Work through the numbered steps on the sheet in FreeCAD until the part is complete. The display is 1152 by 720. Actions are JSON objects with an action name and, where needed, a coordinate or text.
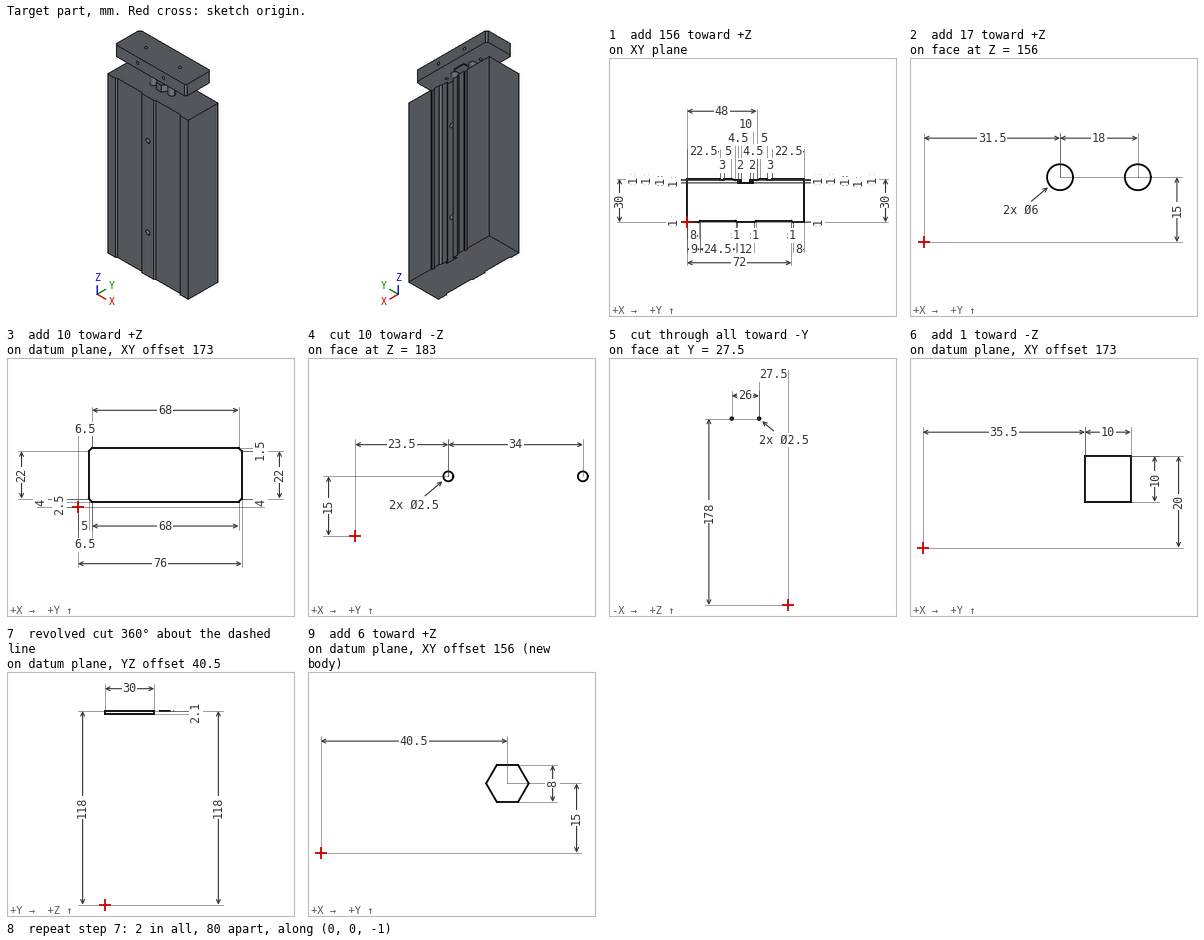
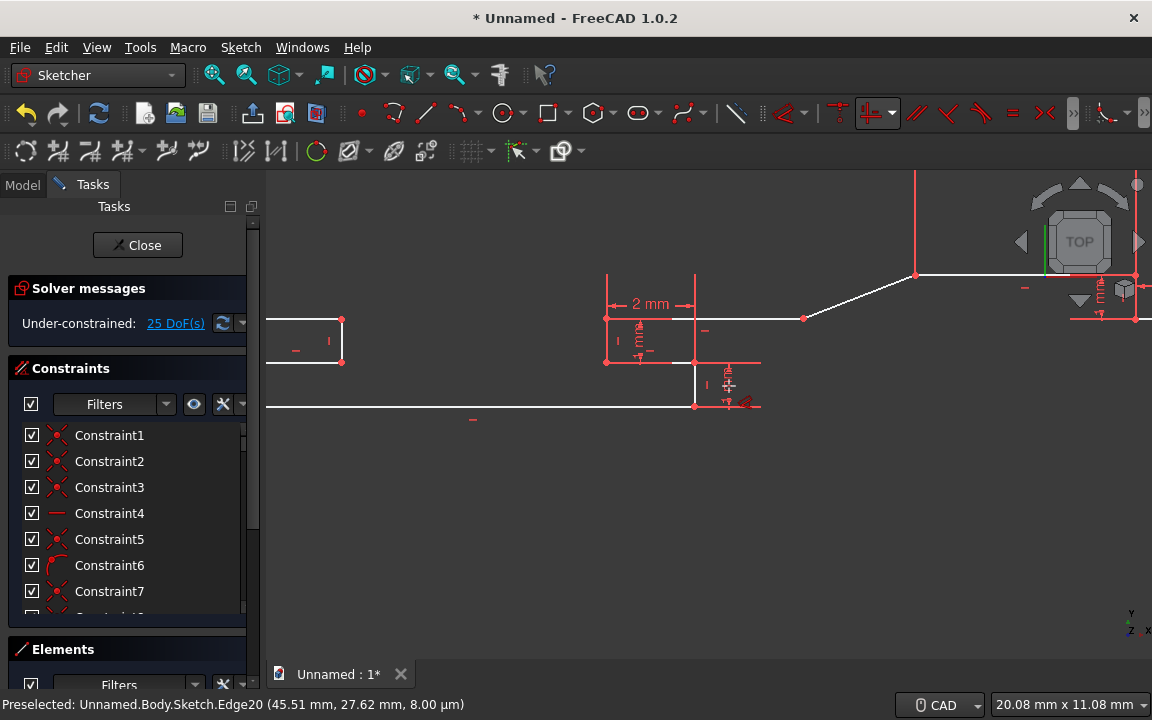
{"action": "scroll", "coordinate": [667, 333], "scroll_direction": "down", "scroll_amount": 10}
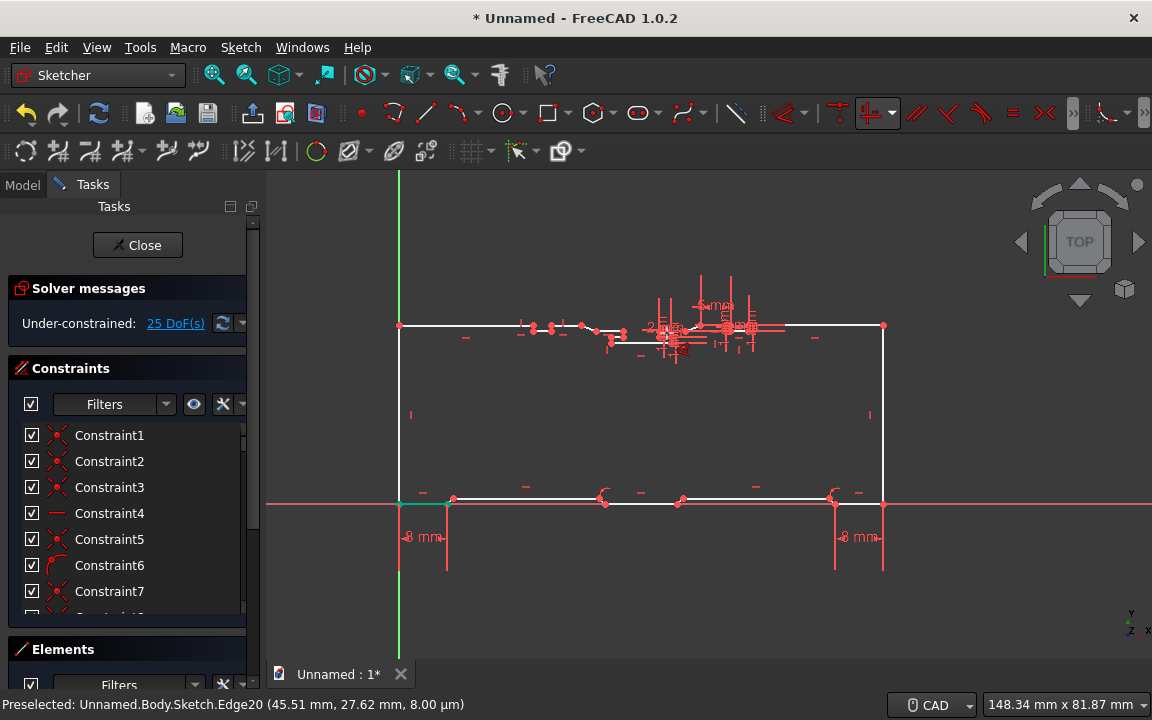
{"action": "scroll", "coordinate": [611, 341], "scroll_direction": "up", "scroll_amount": 11}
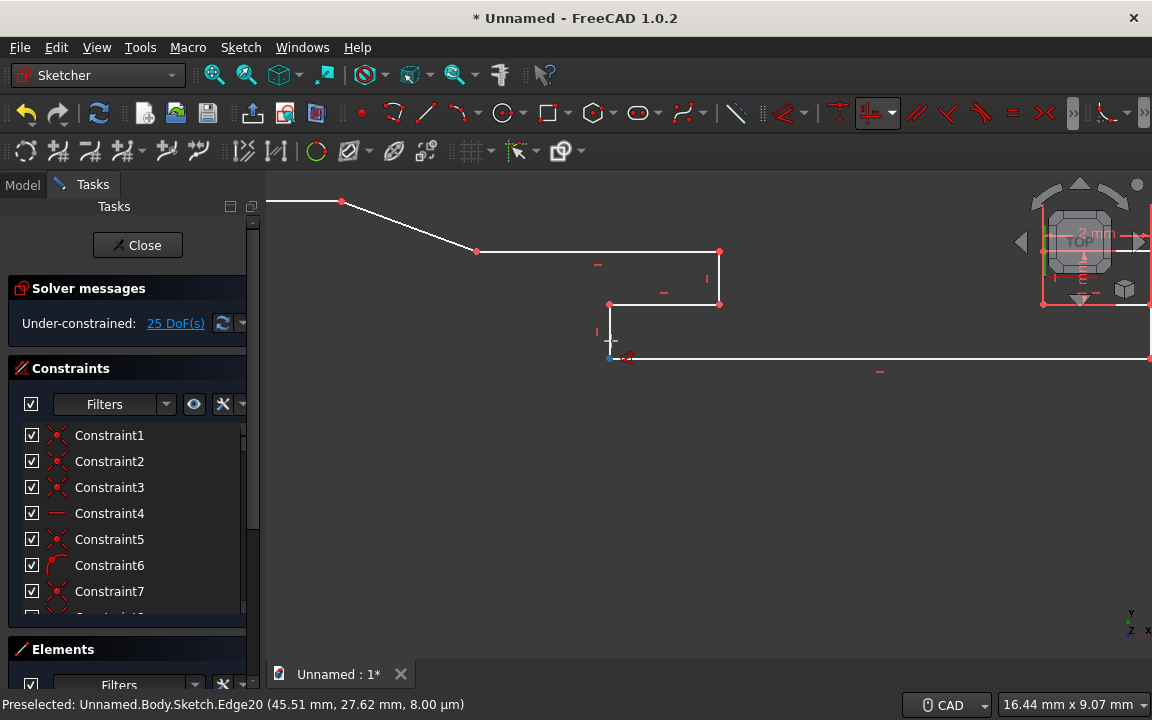
{"action": "left_click", "coordinate": [610, 343]}
{"action": "left_click", "coordinate": [576, 332]}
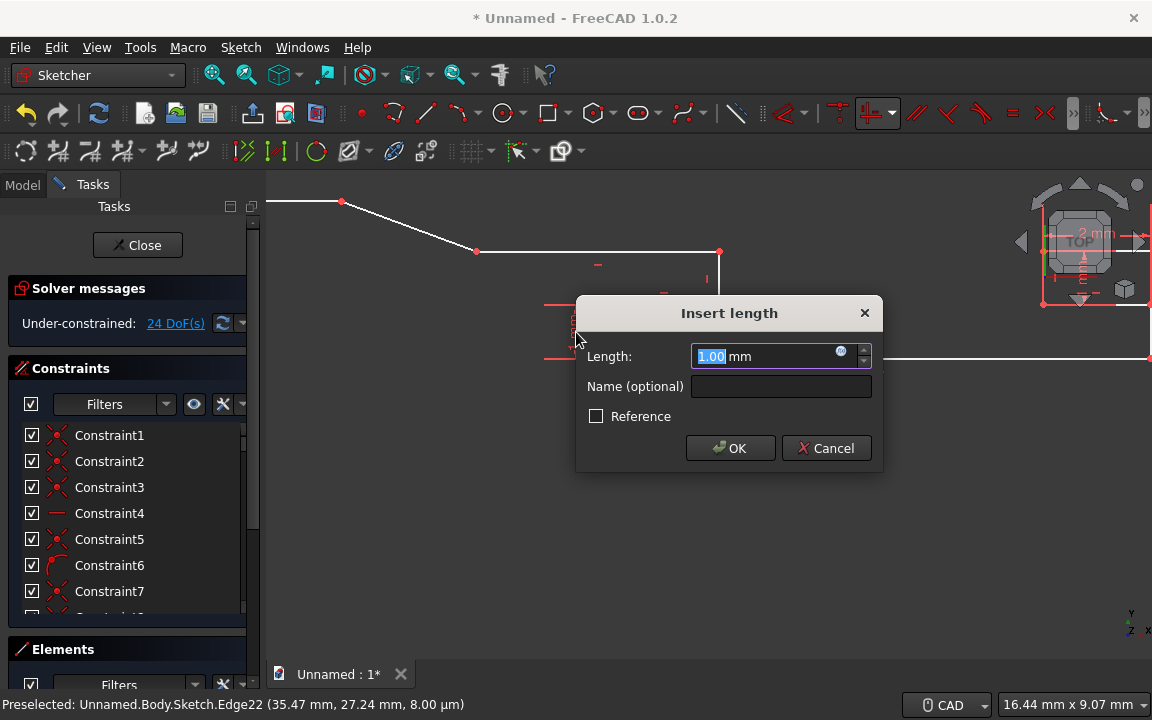
{"action": "type", "text": "1"}
{"action": "key", "text": "Return"}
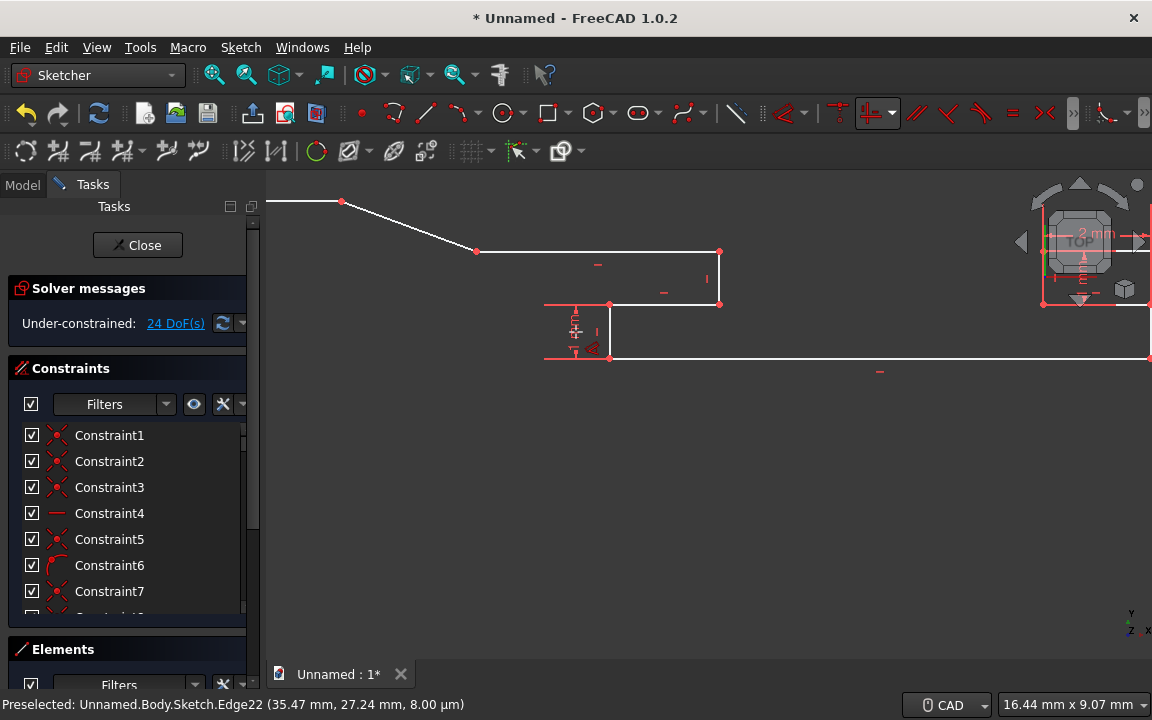
{"action": "left_click", "coordinate": [643, 305]}
{"action": "left_click", "coordinate": [664, 271]}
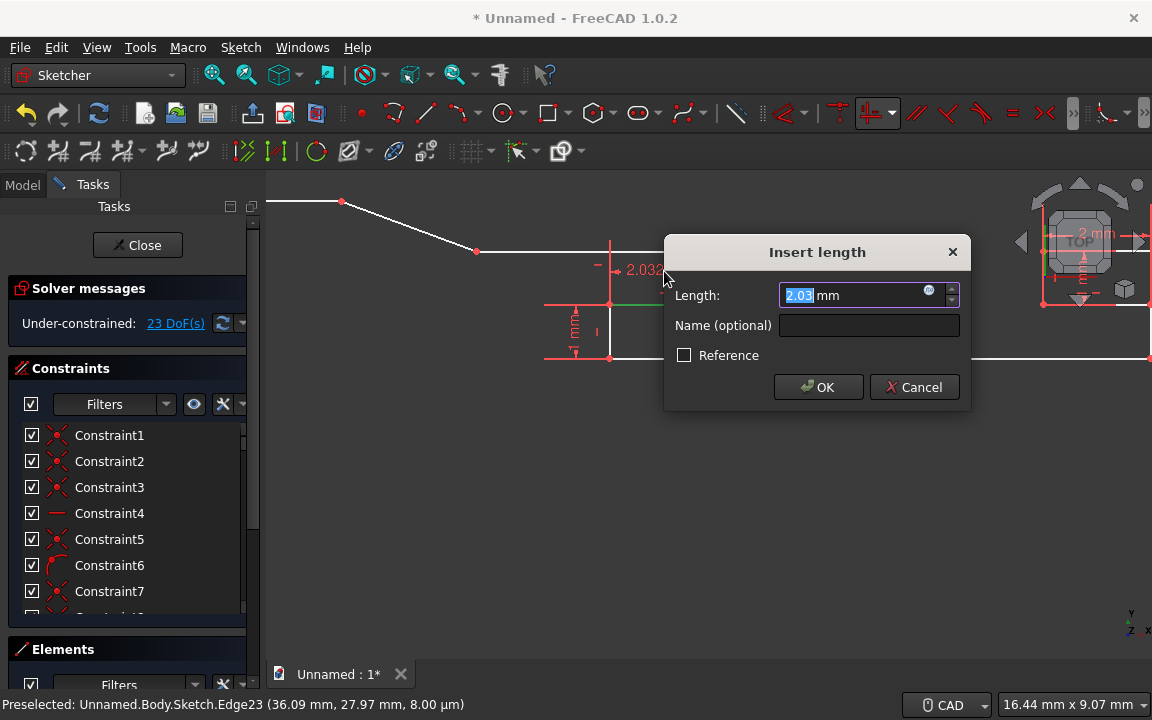
{"action": "type", "text": "2"}
{"action": "key", "text": "Return"}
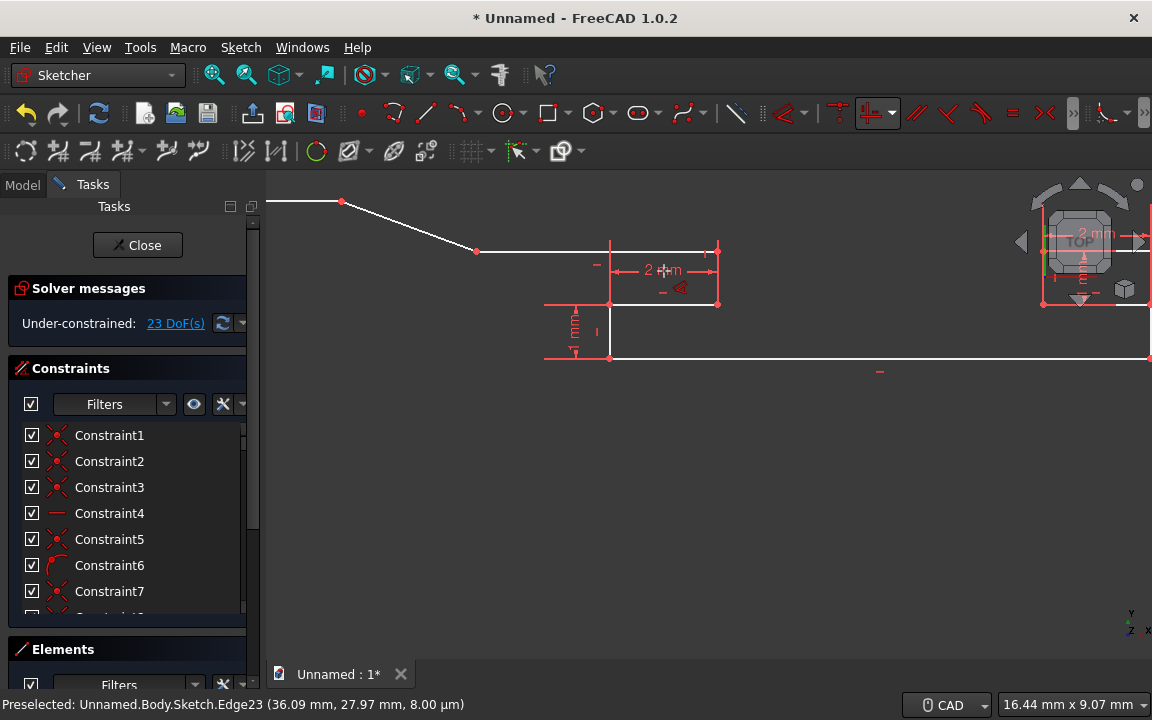
{"action": "left_click", "coordinate": [718, 289]}
{"action": "left_click", "coordinate": [752, 278]}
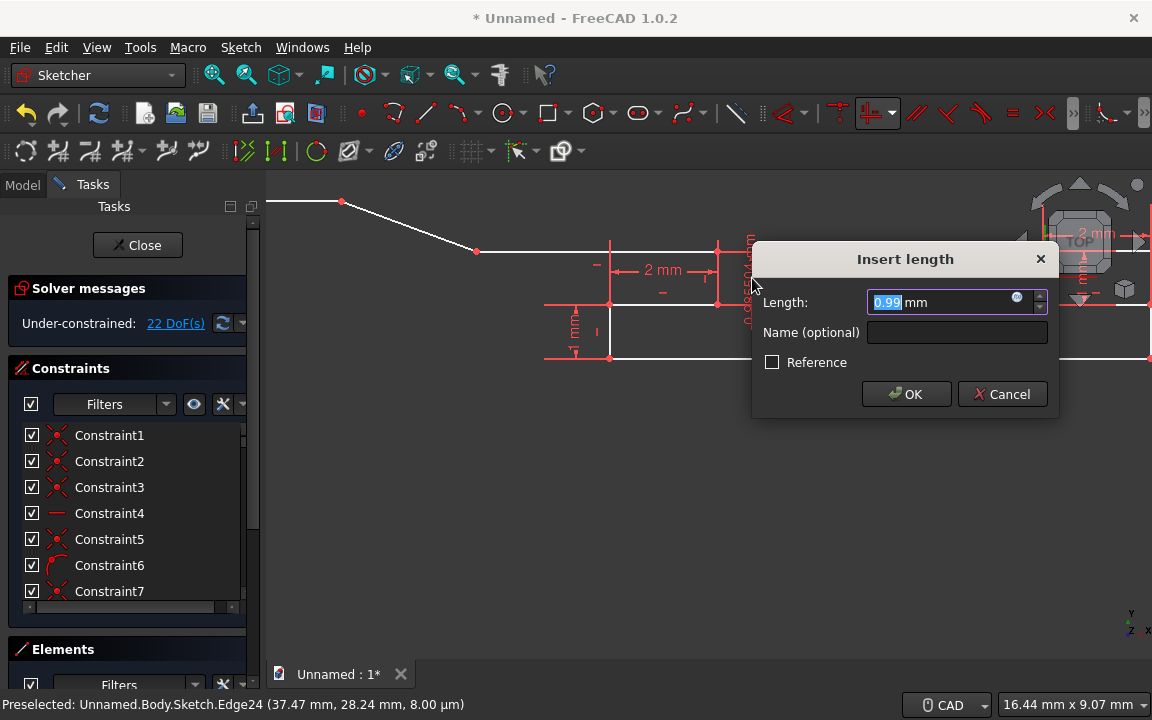
{"action": "type", "text": "1"}
{"action": "key", "text": "Return"}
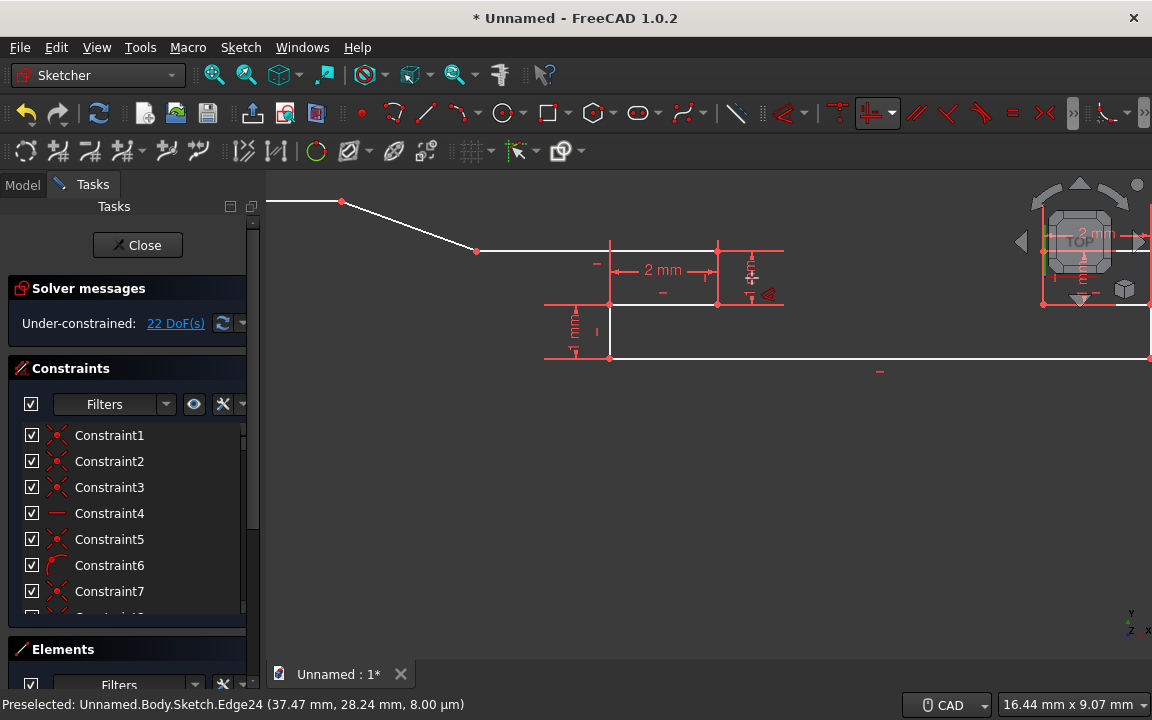
{"action": "scroll", "coordinate": [611, 341], "scroll_direction": "down", "scroll_amount": 11}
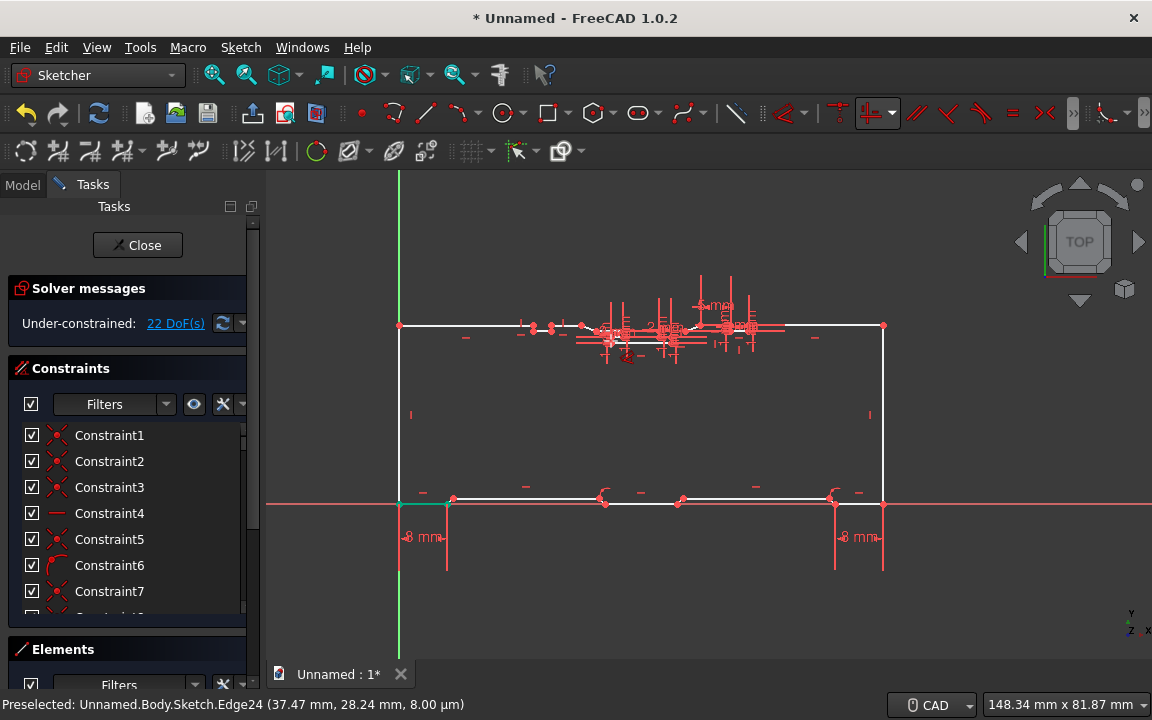
{"action": "scroll", "coordinate": [572, 326], "scroll_direction": "up", "scroll_amount": 3}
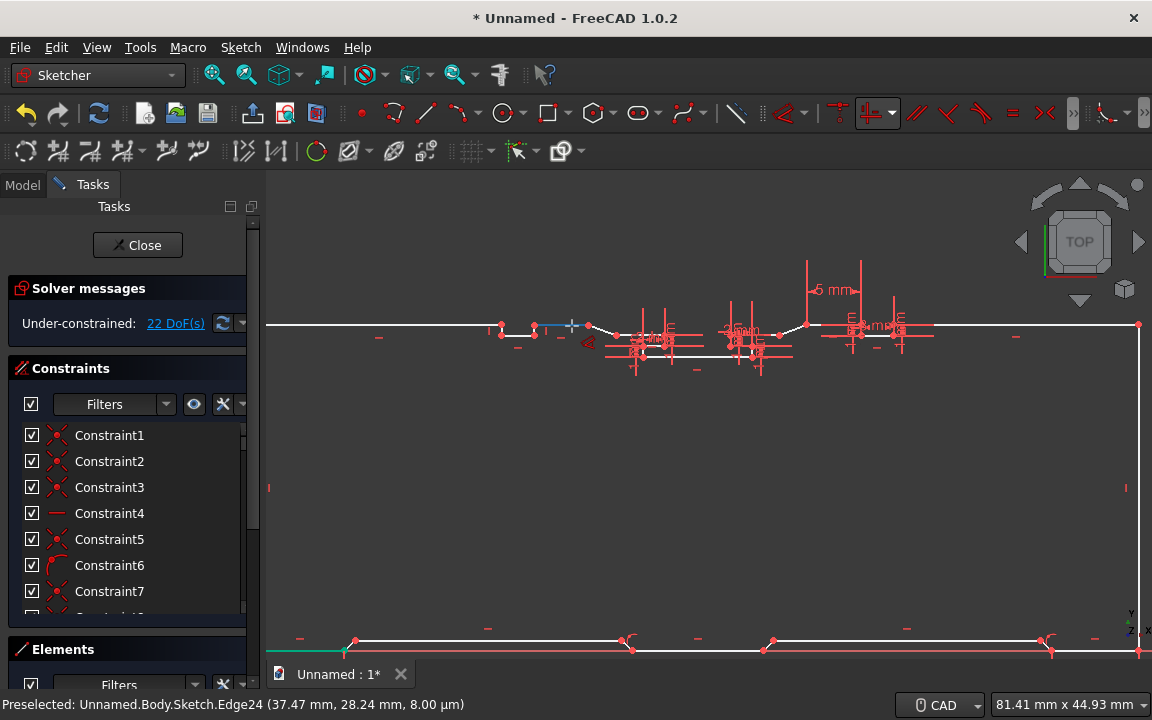
{"action": "left_click", "coordinate": [573, 325]}
{"action": "left_click", "coordinate": [562, 291]}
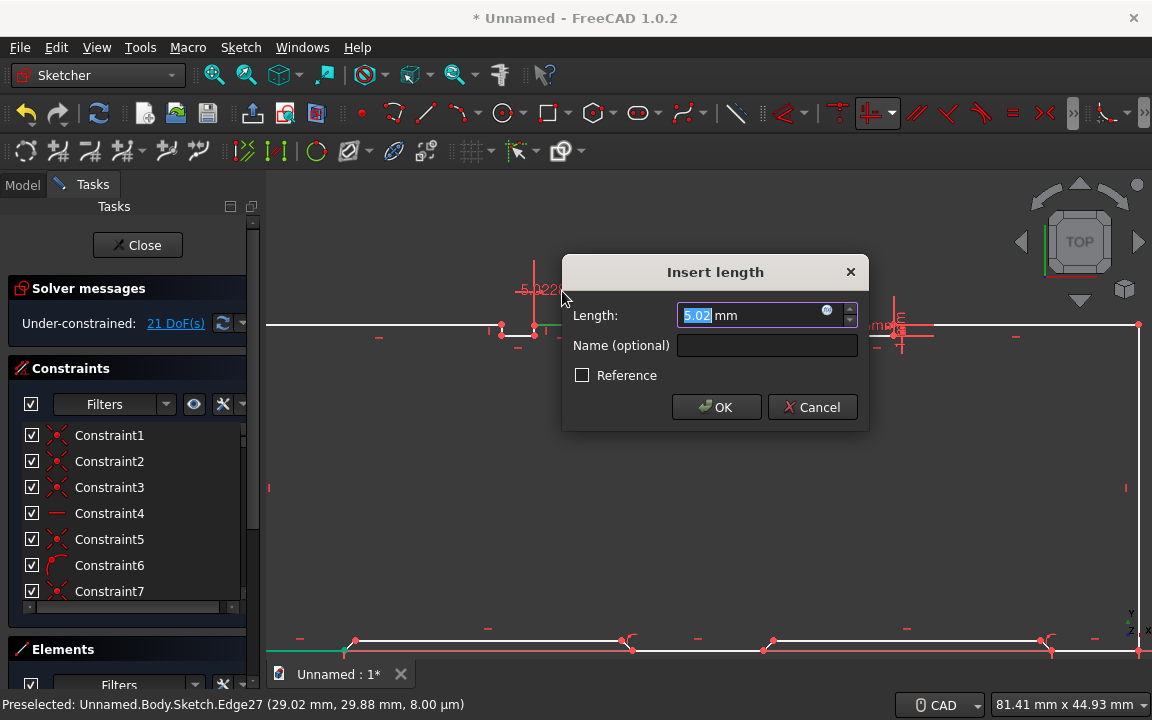
{"action": "type", "text": "5"}
{"action": "key", "text": "Return"}